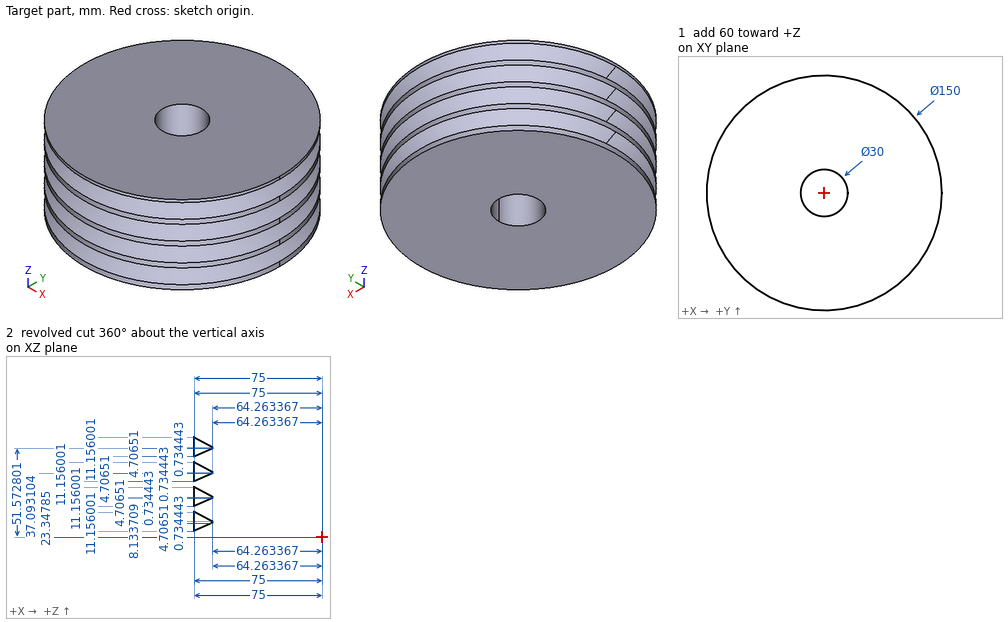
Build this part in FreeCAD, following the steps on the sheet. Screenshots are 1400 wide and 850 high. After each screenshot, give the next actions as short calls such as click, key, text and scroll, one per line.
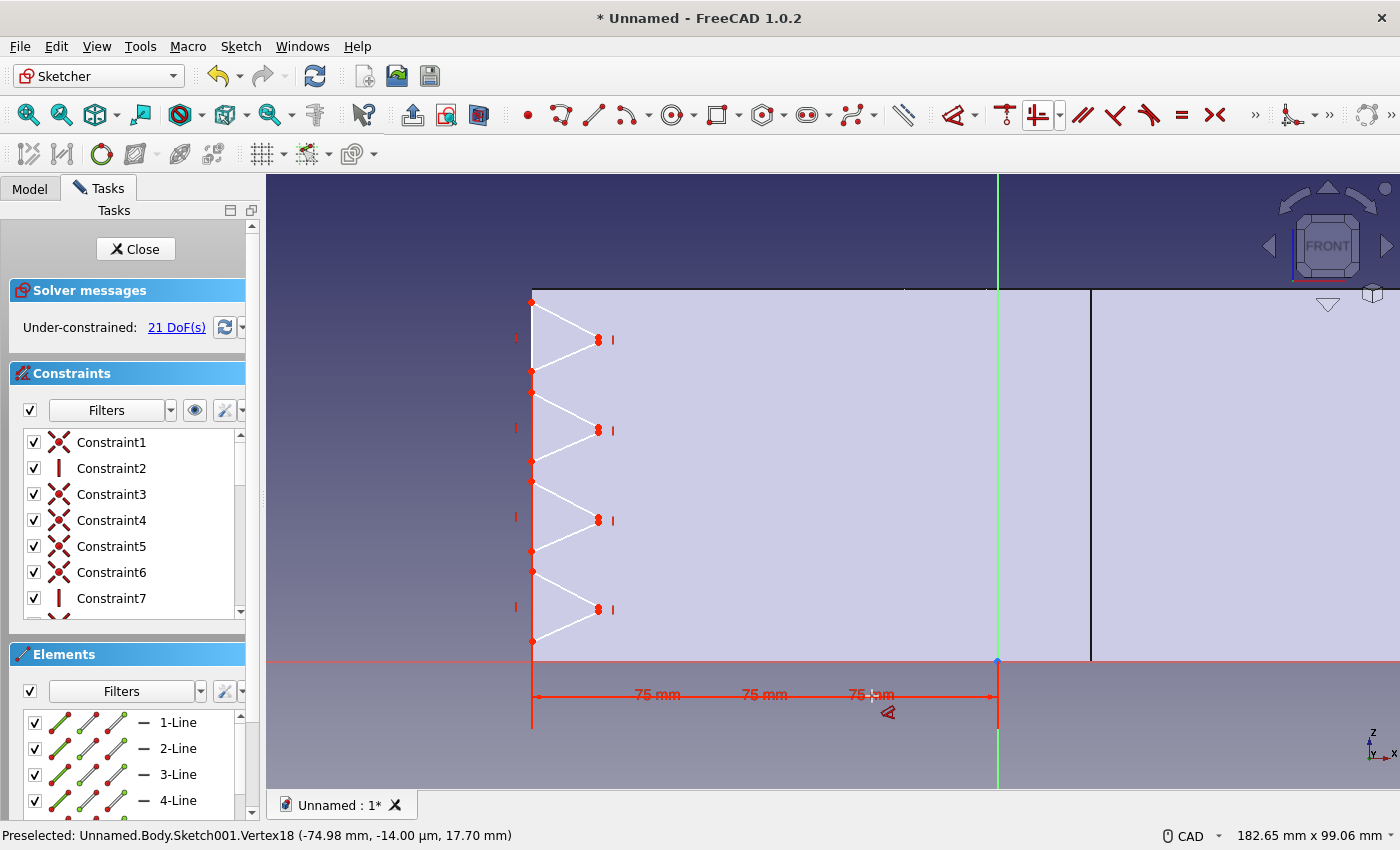
click(532, 642)
click(765, 608)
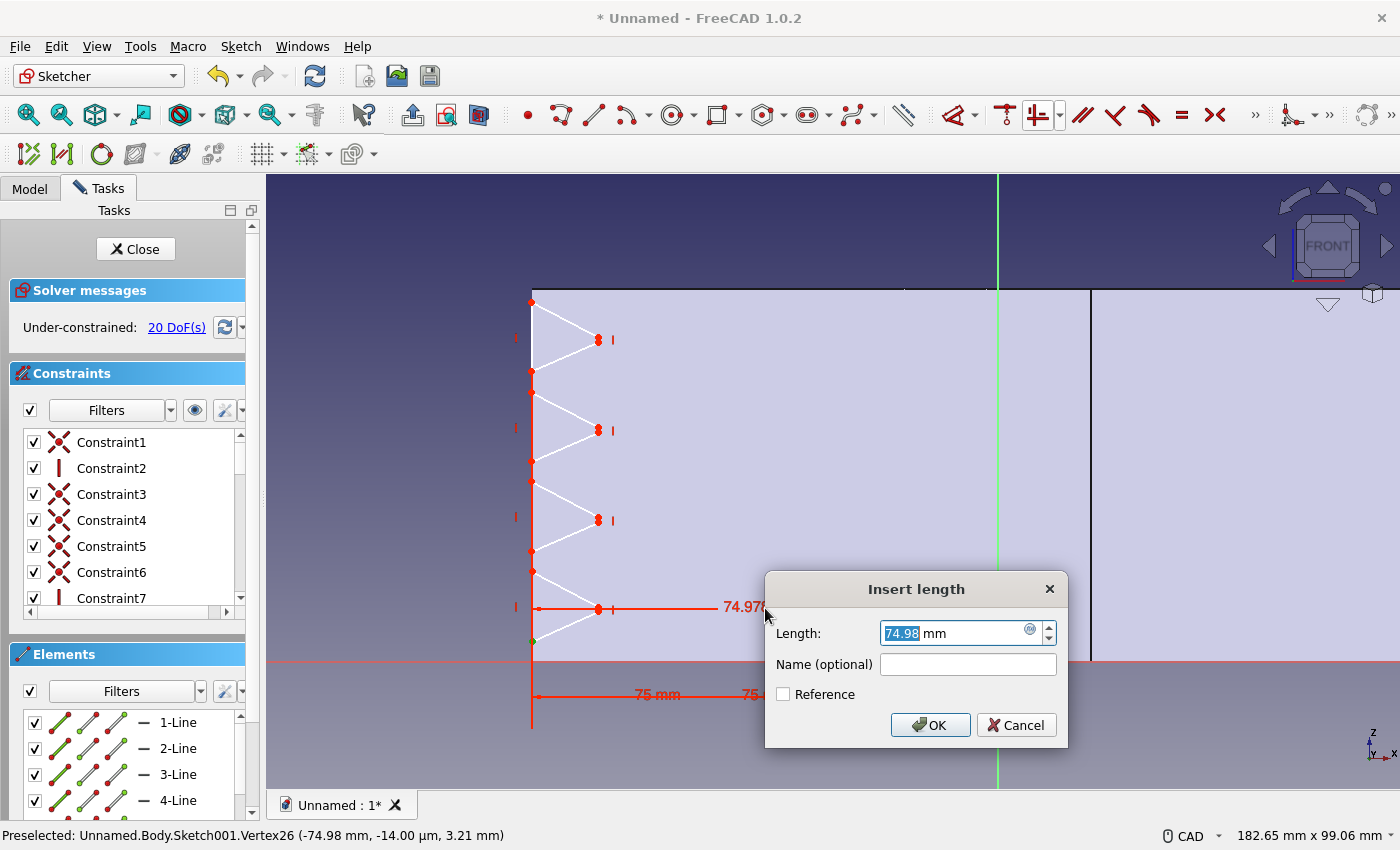
text(75)
key(Return)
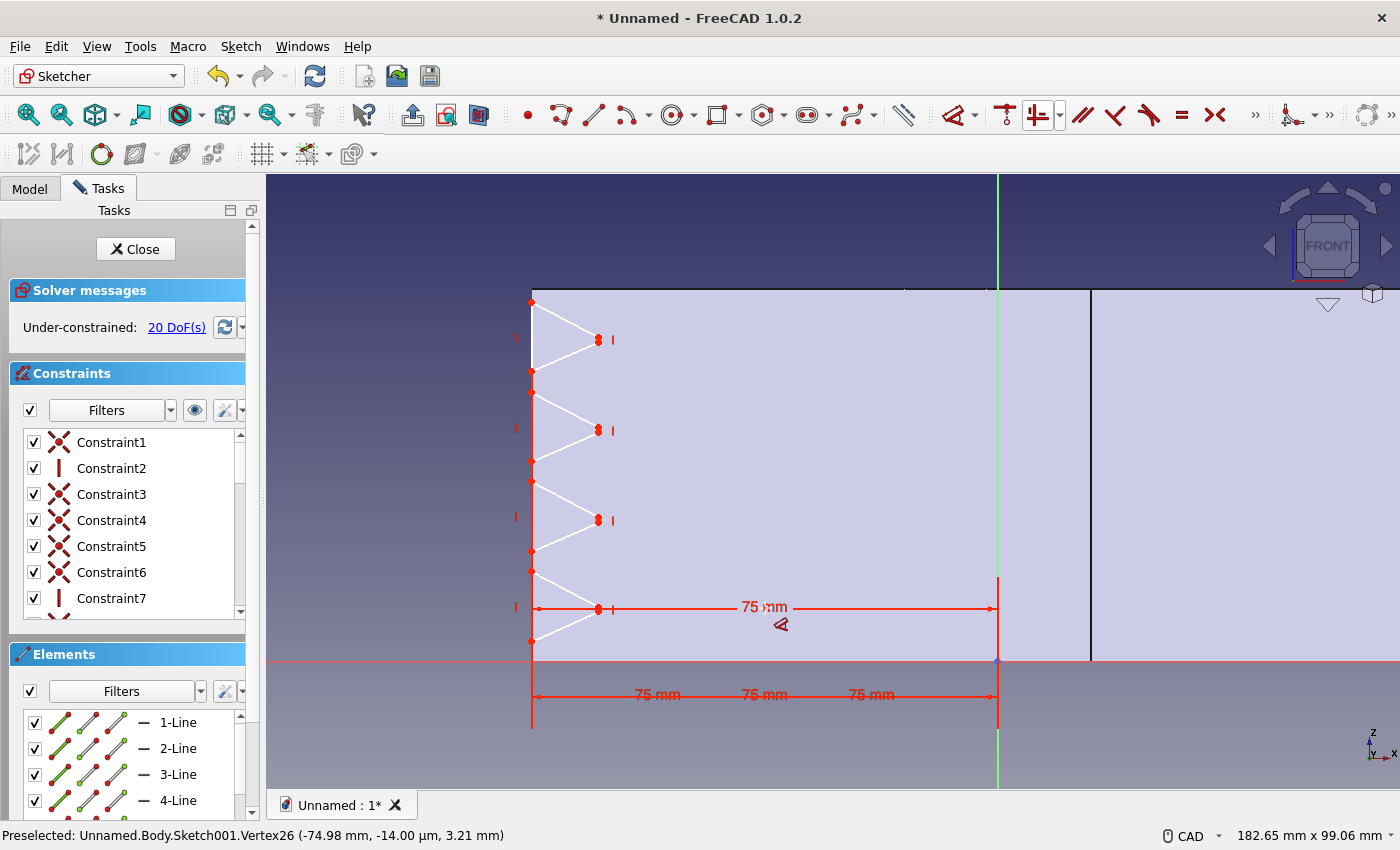
scroll(598, 340, up, 11)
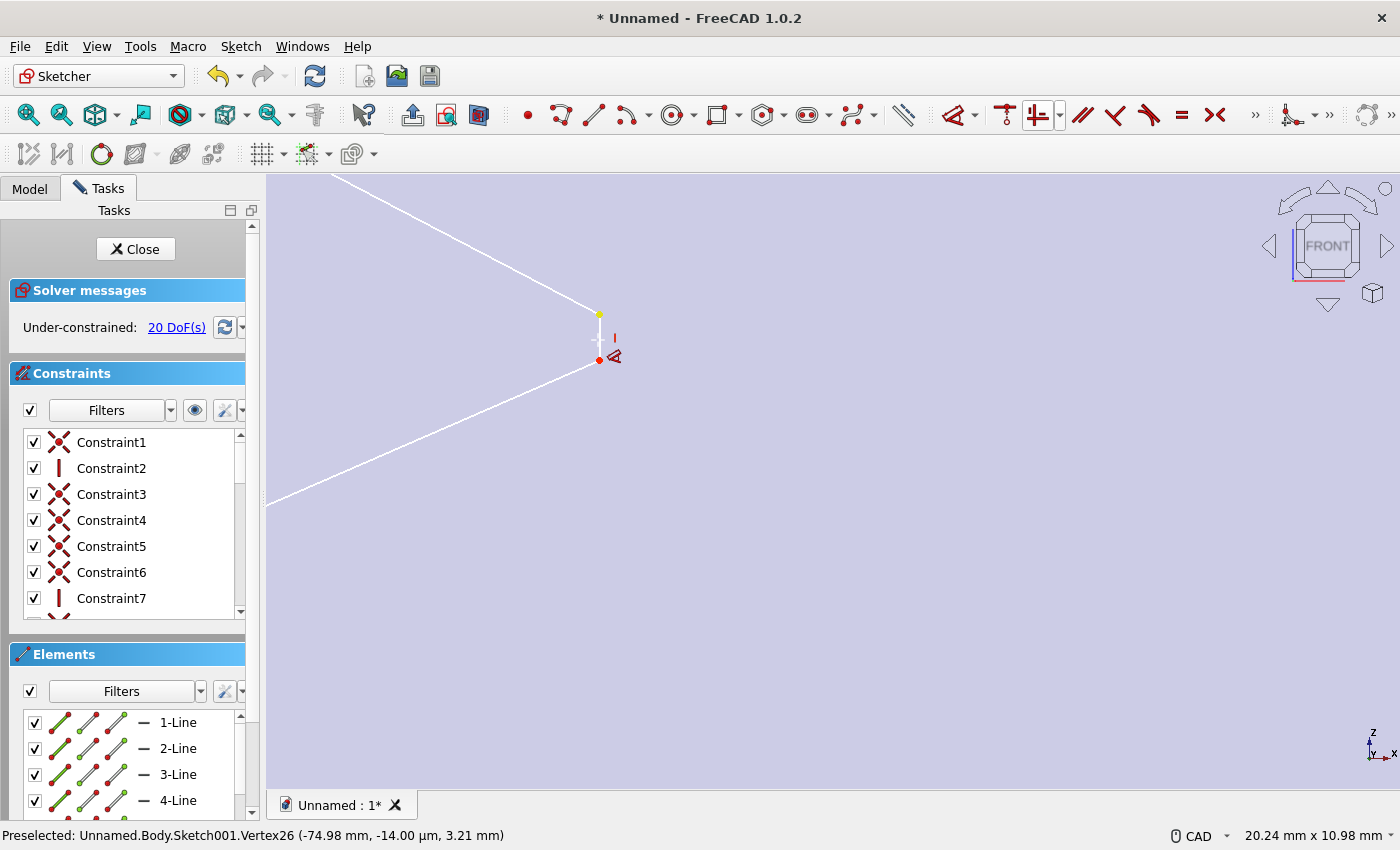
click(600, 338)
click(566, 338)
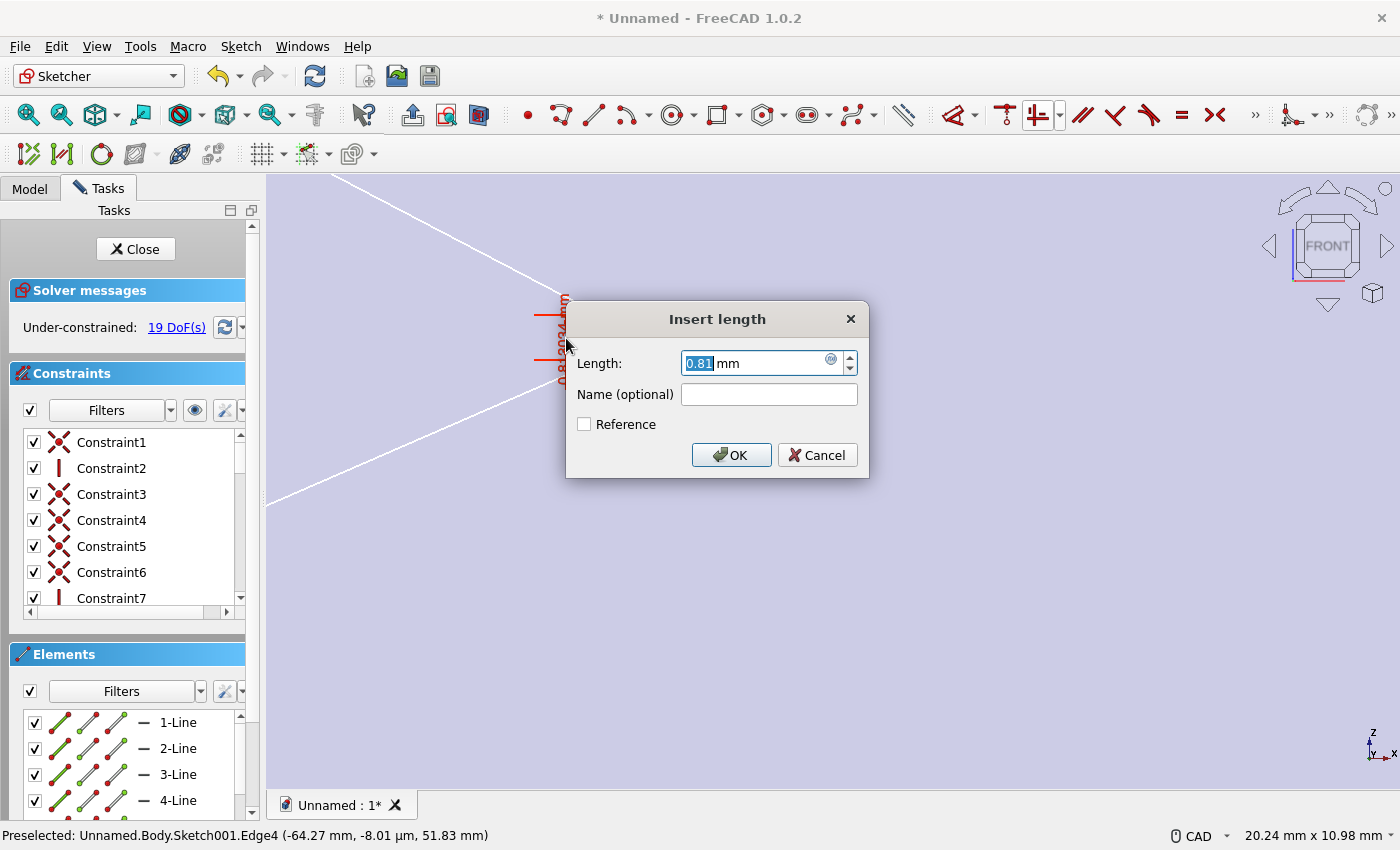
text(0.734443)
key(Return)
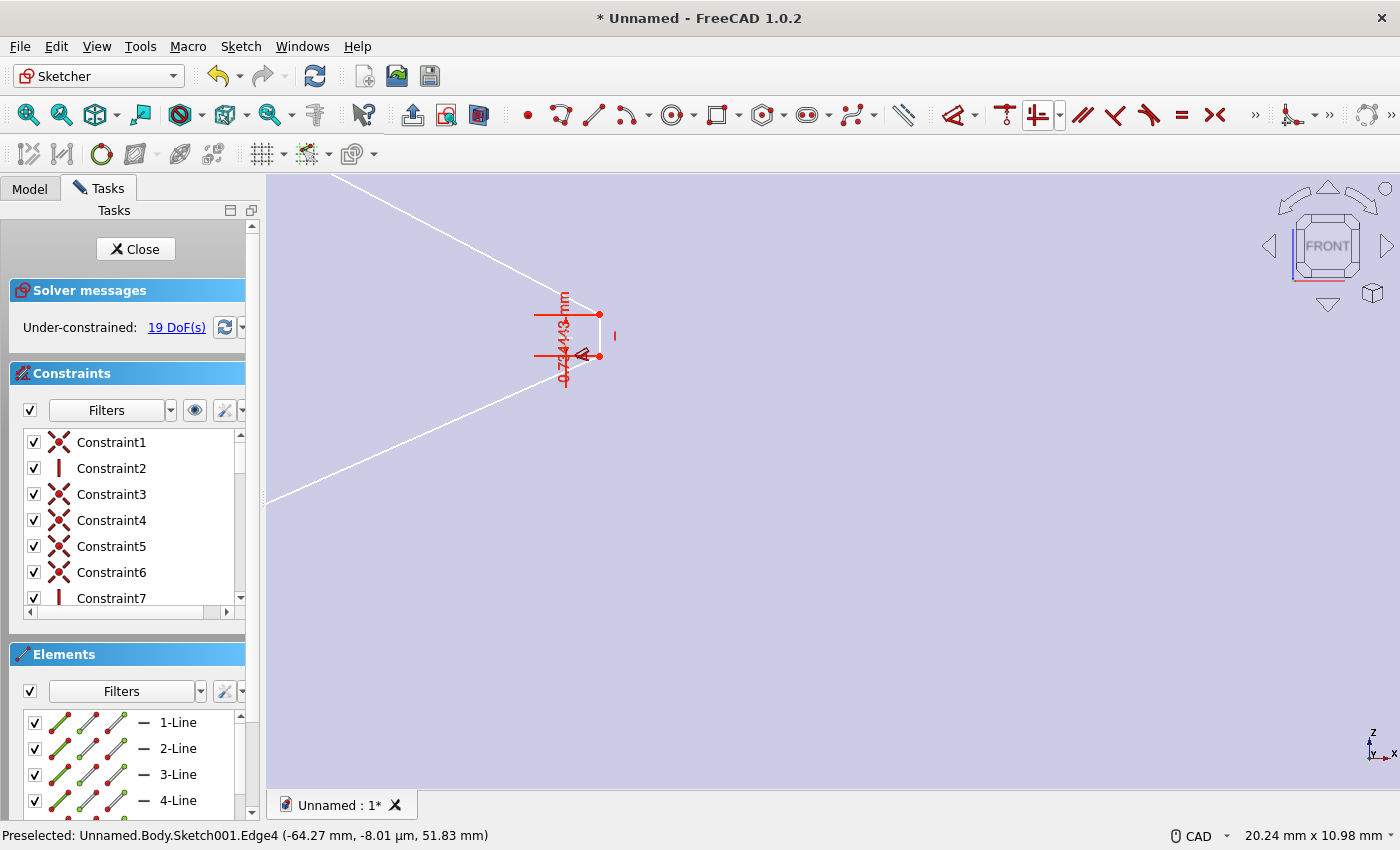
scroll(598, 340, down, 11)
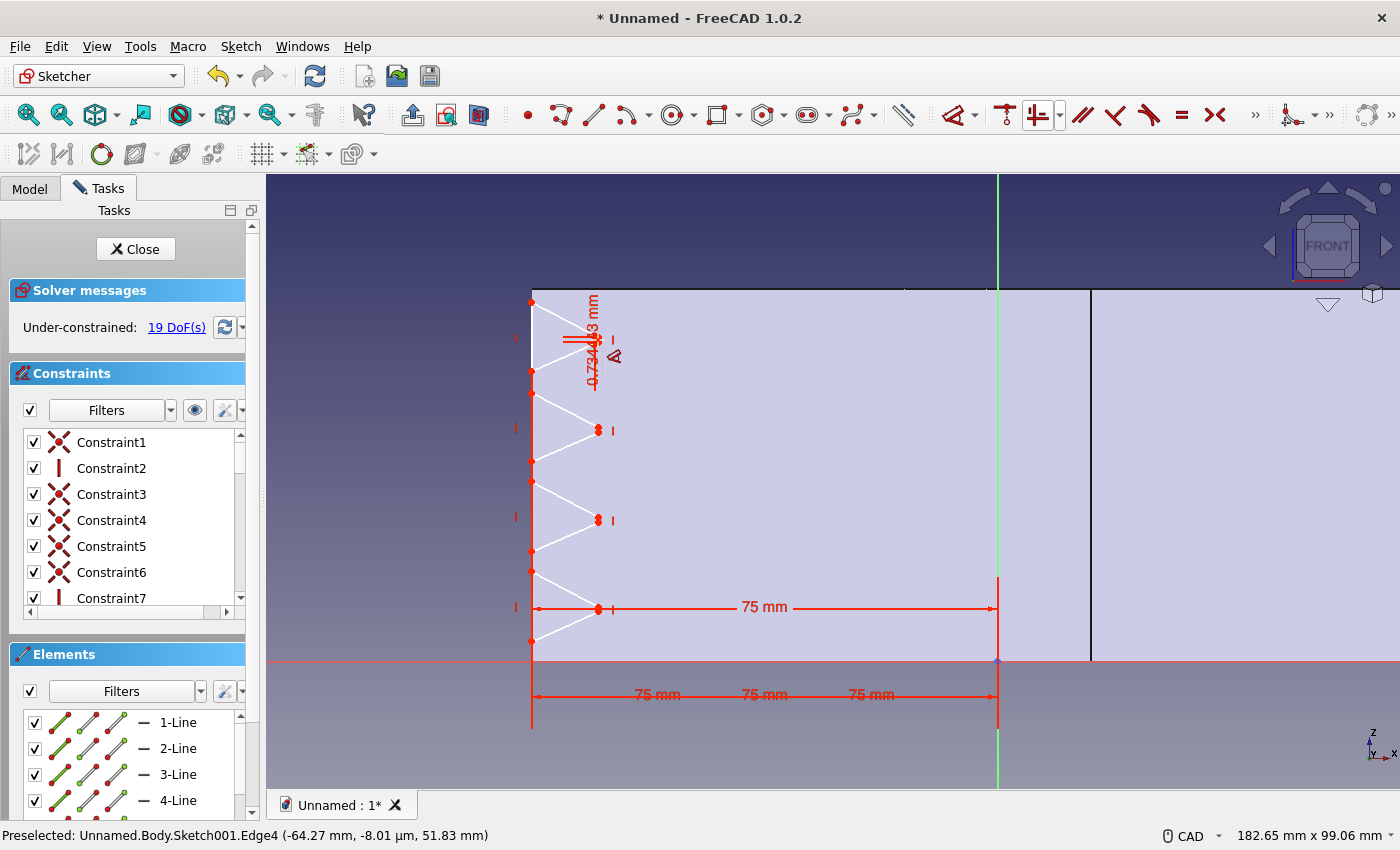
scroll(598, 429, up, 11)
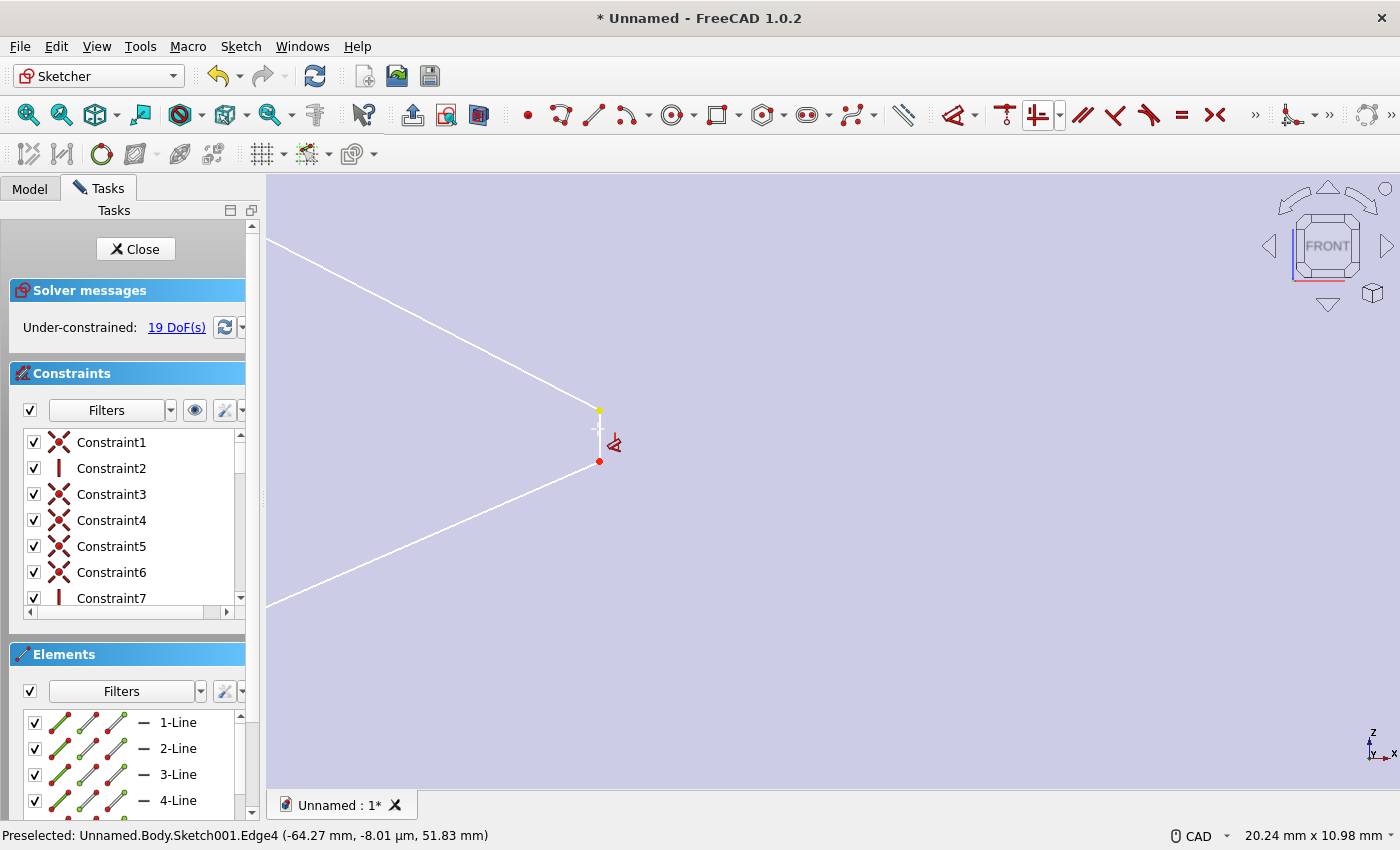
click(600, 426)
click(566, 436)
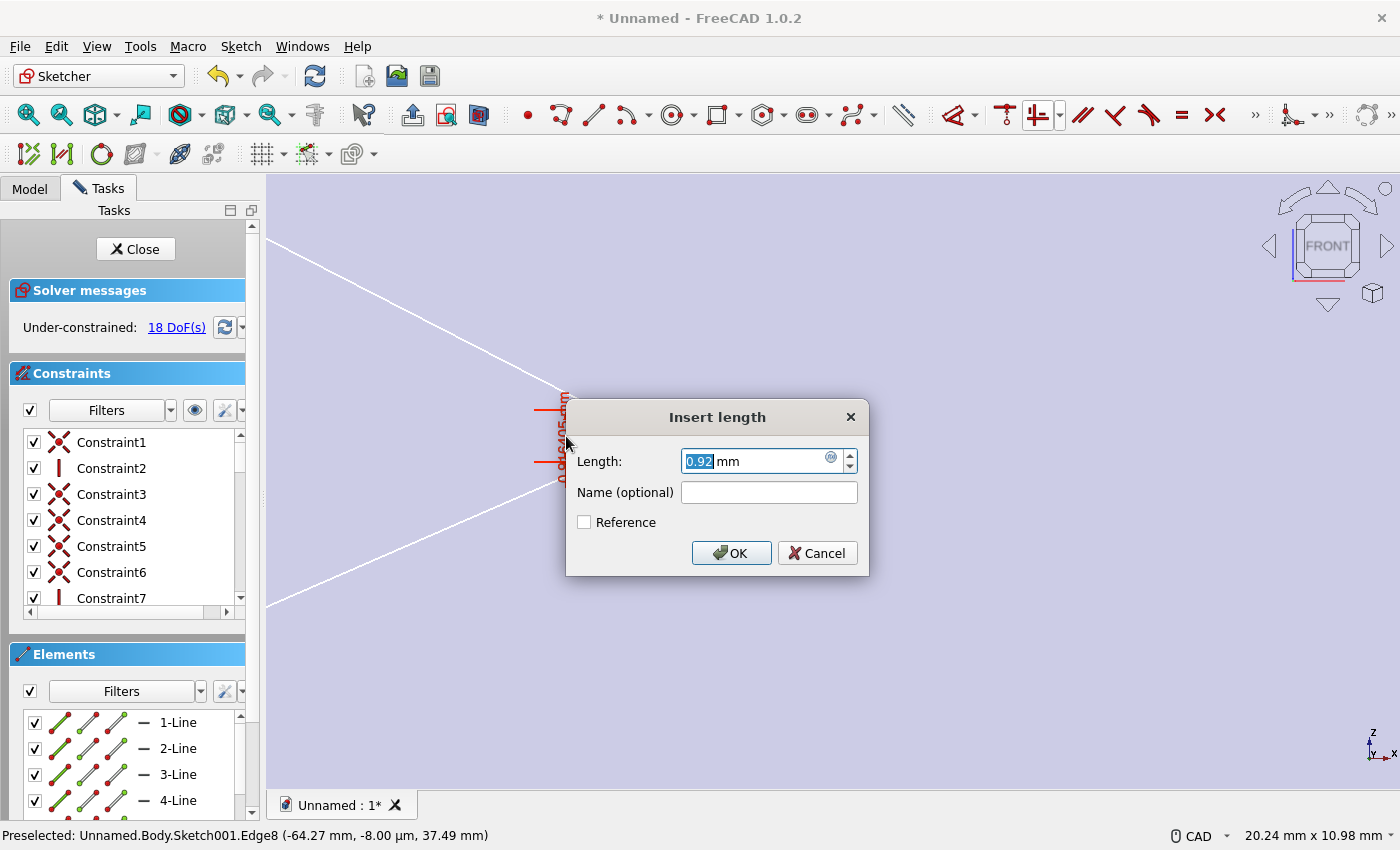
text(0.734443)
key(Return)